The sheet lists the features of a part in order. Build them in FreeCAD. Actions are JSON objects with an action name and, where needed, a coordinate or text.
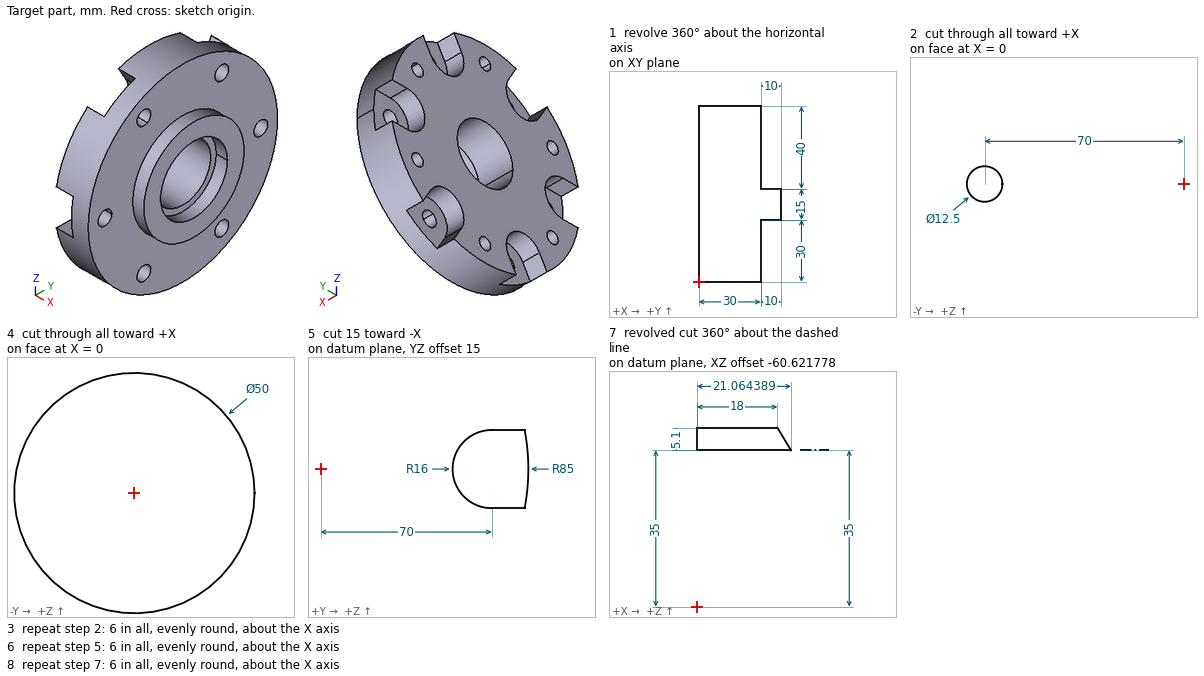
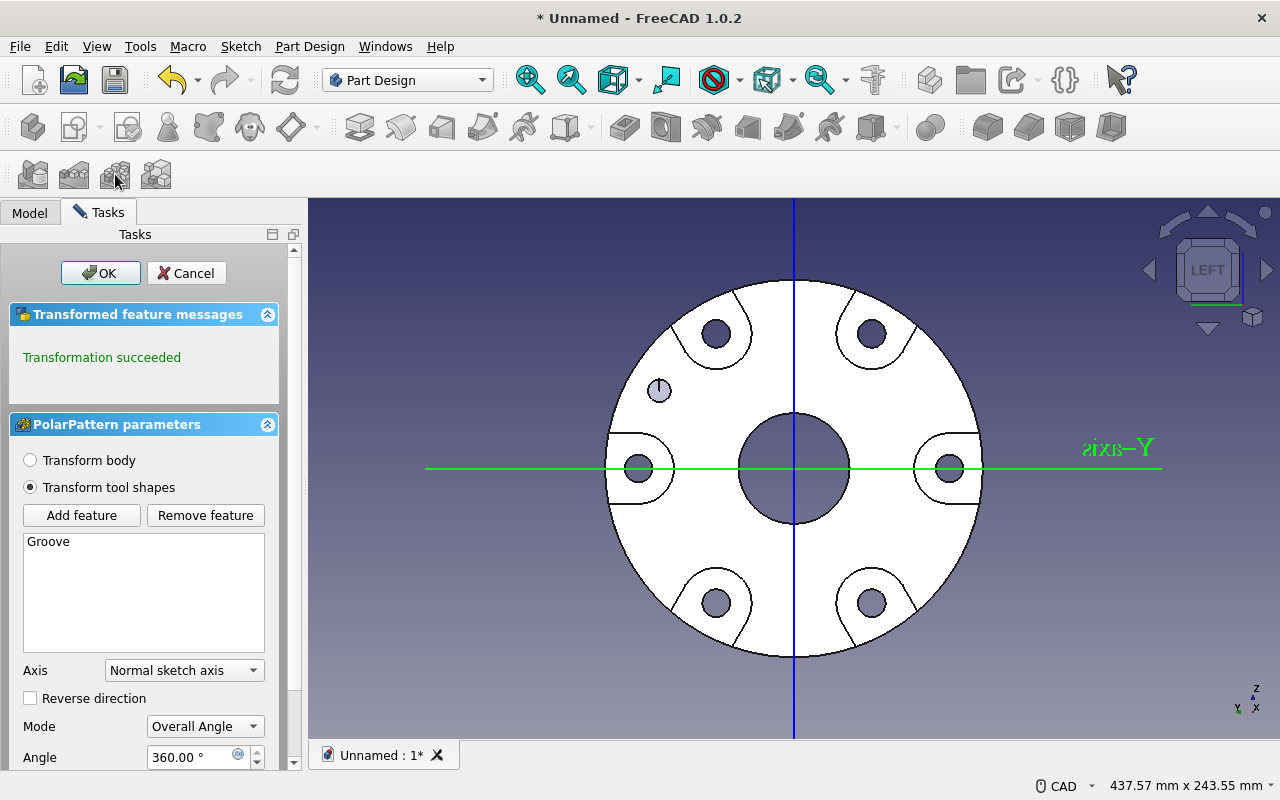
{"action": "left_click", "coordinate": [185, 670]}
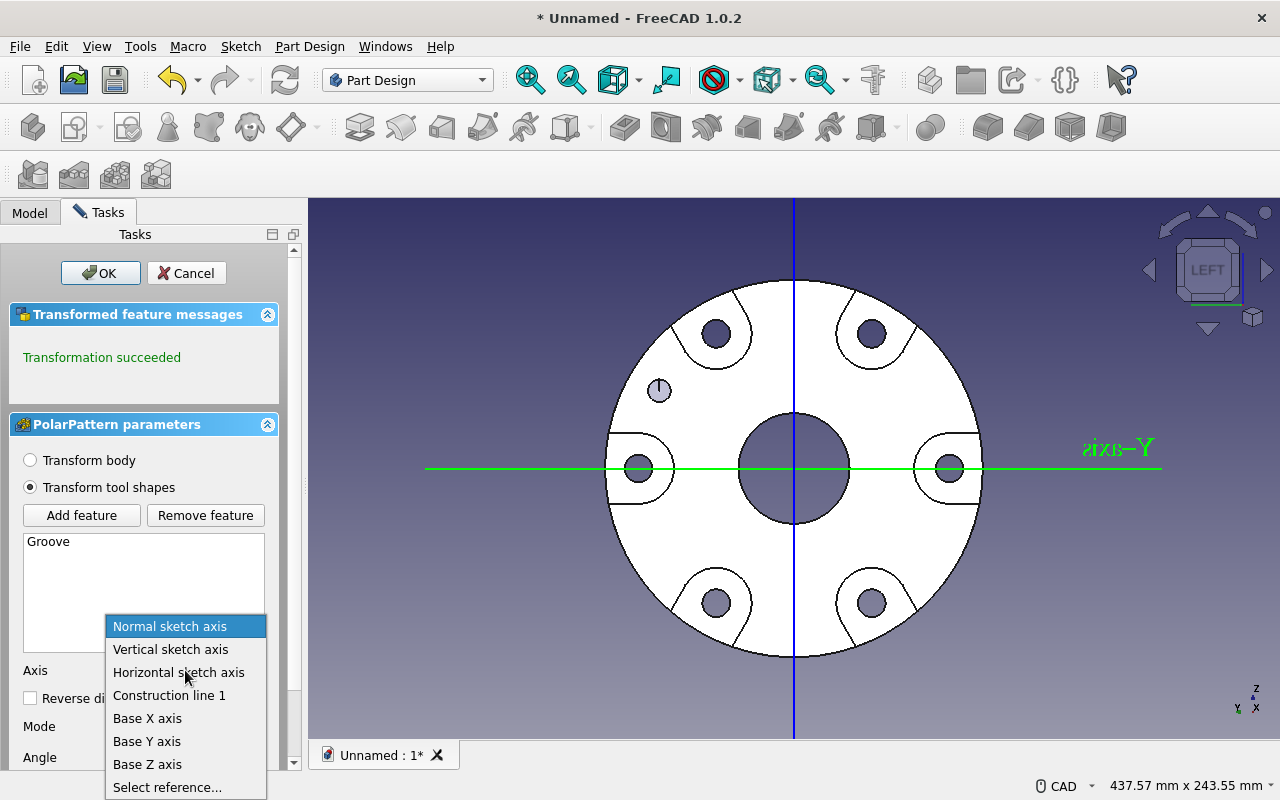
{"action": "left_click", "coordinate": [184, 718]}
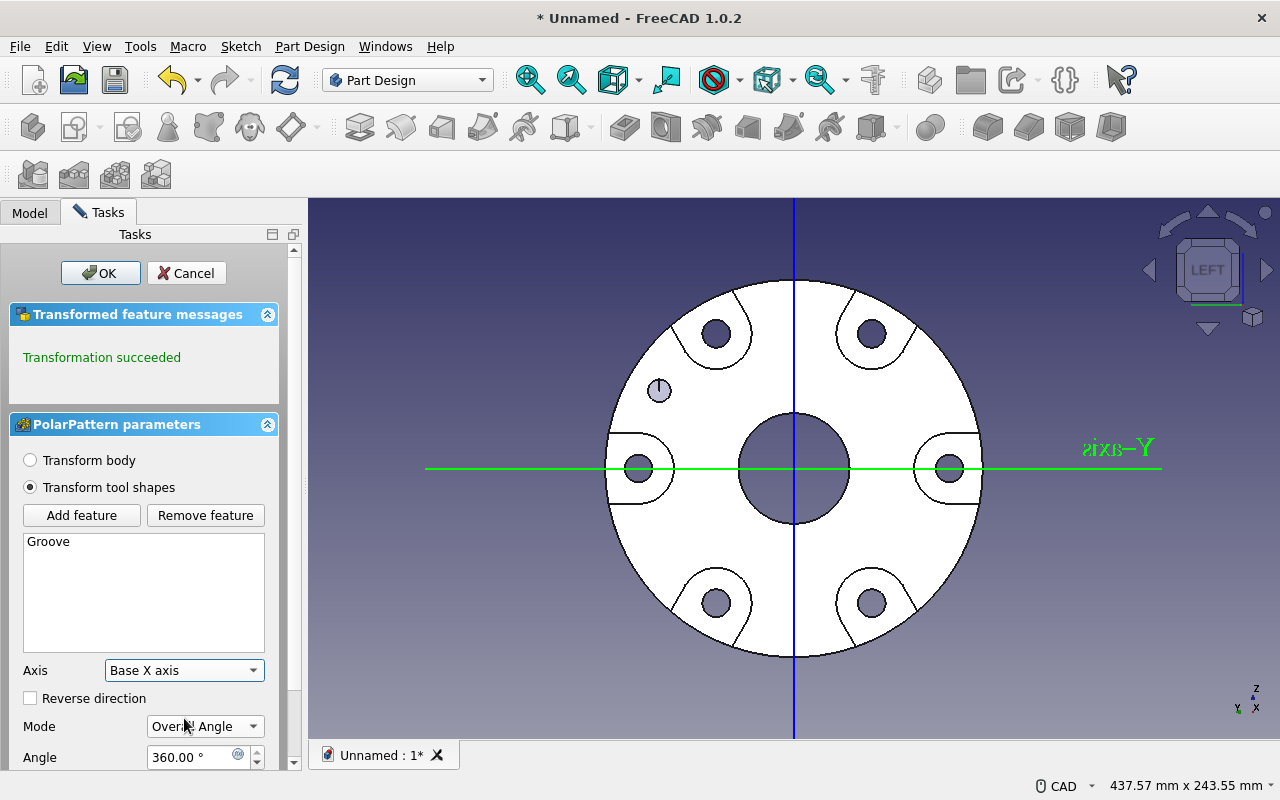
{"action": "scroll", "coordinate": [294, 507], "scroll_direction": "down", "scroll_amount": 2}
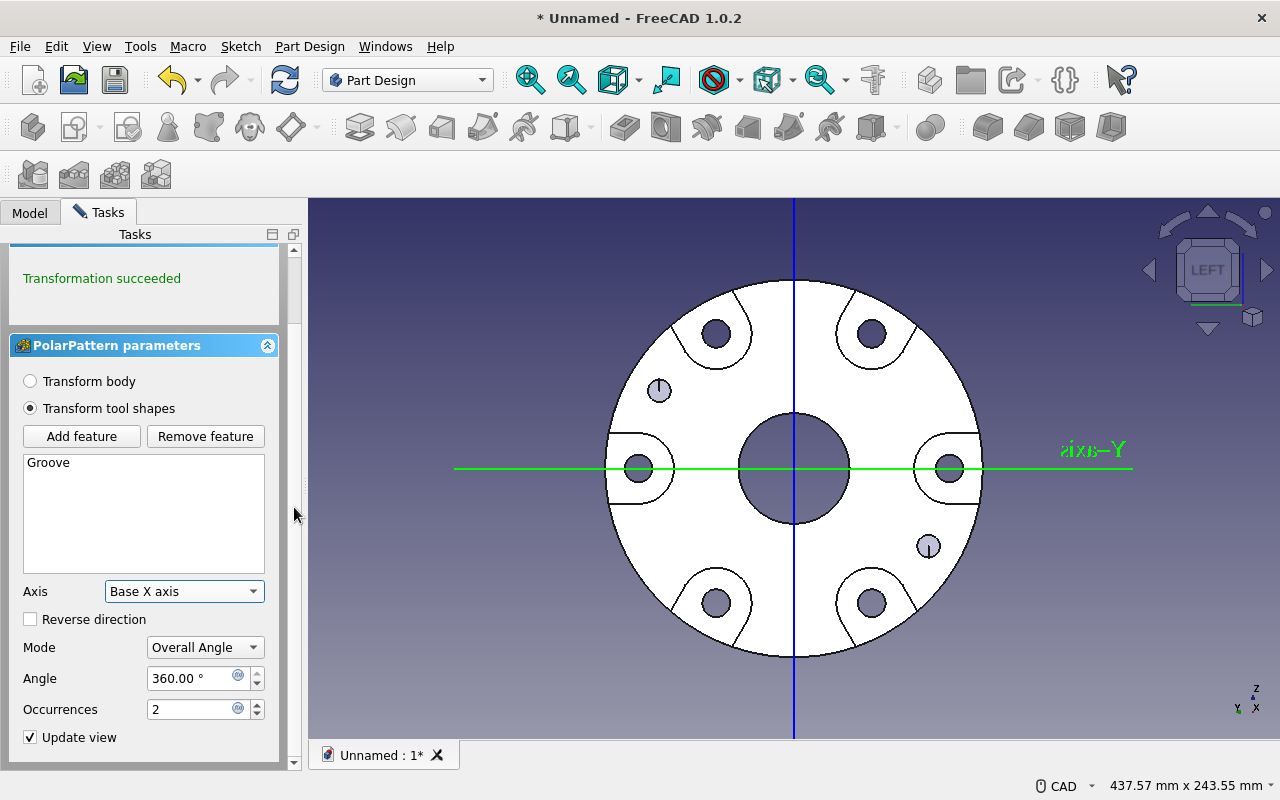
{"action": "triple_click", "coordinate": [199, 710]}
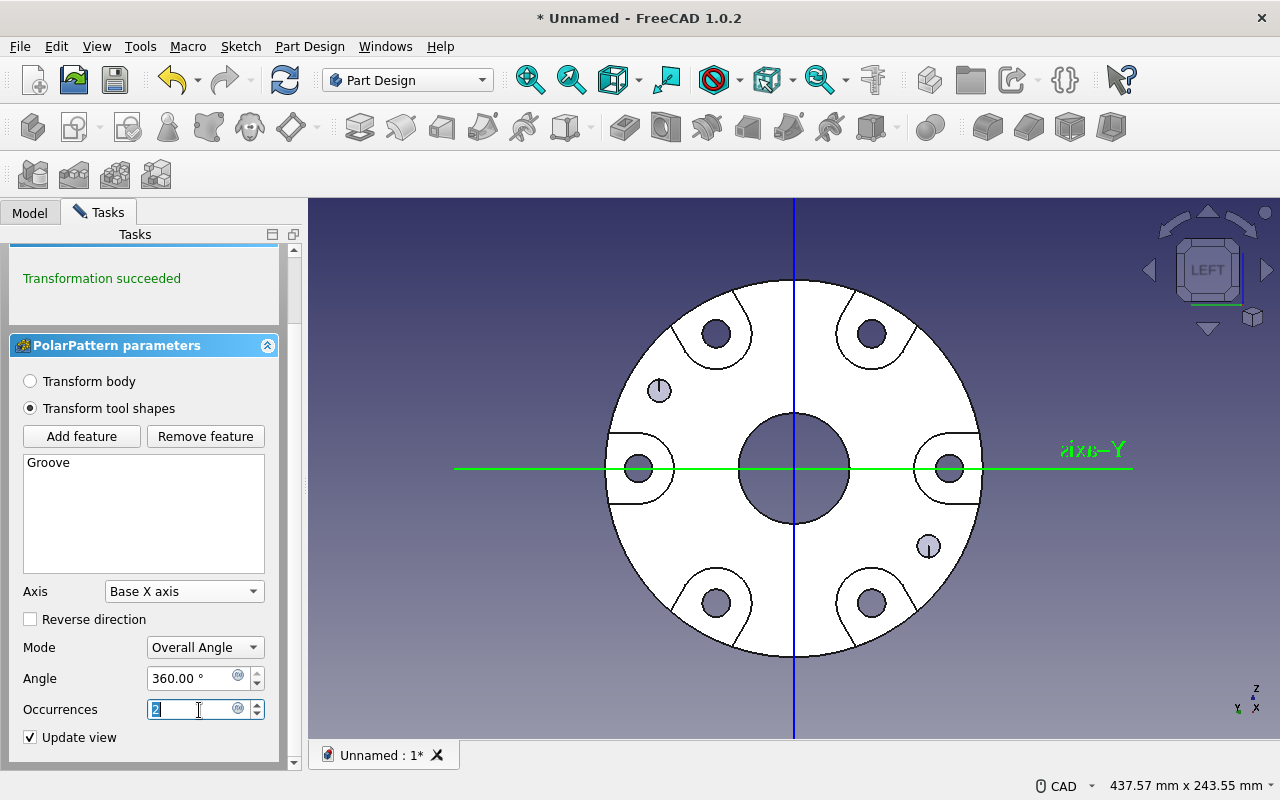
{"action": "type", "text": "6"}
{"action": "key", "text": "Tab"}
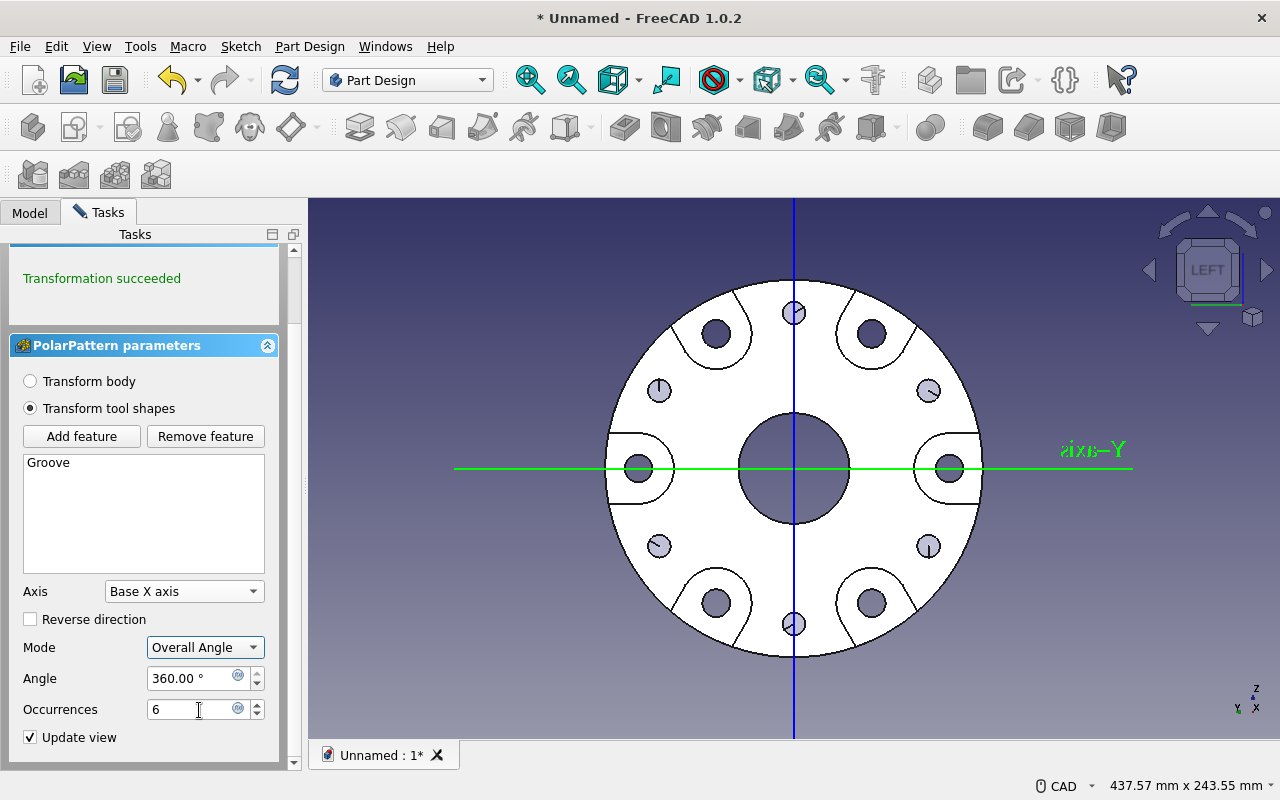
{"action": "scroll", "coordinate": [294, 507], "scroll_direction": "up", "scroll_amount": 3}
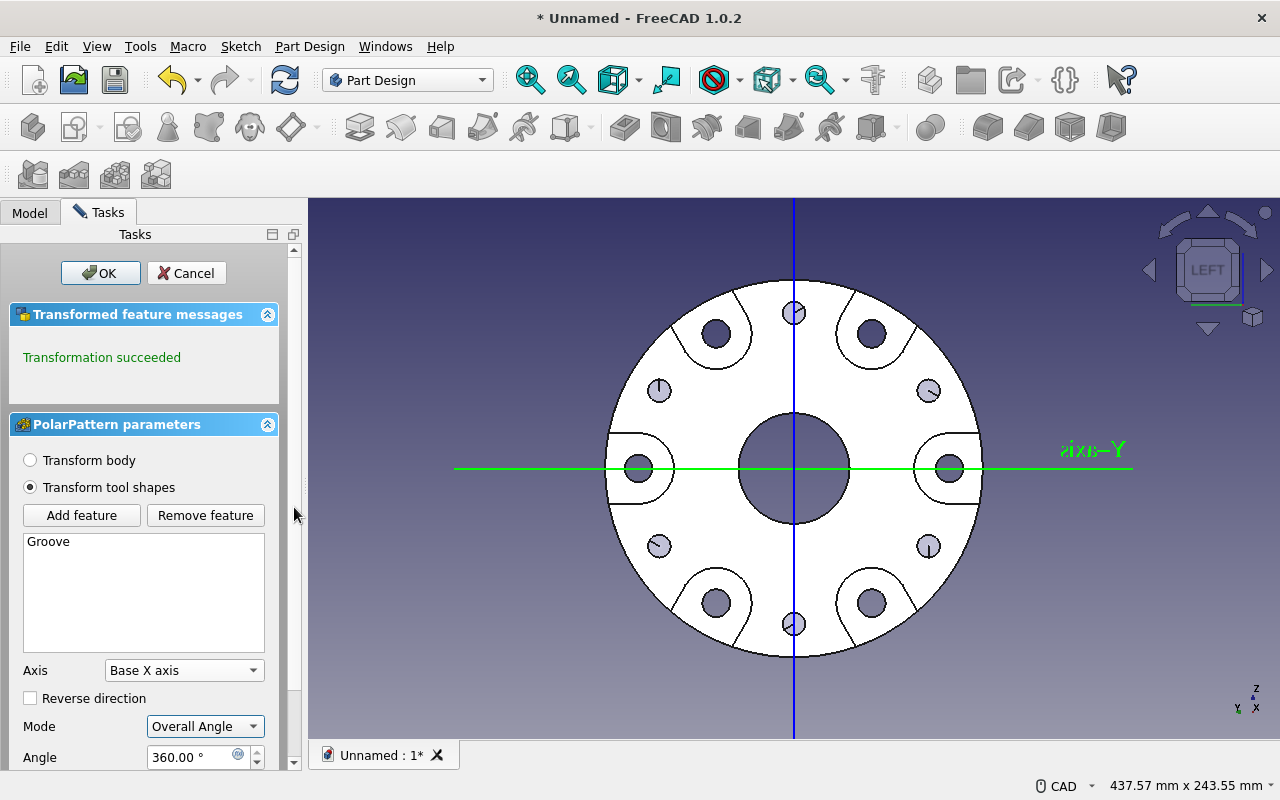
{"action": "left_click", "coordinate": [101, 273]}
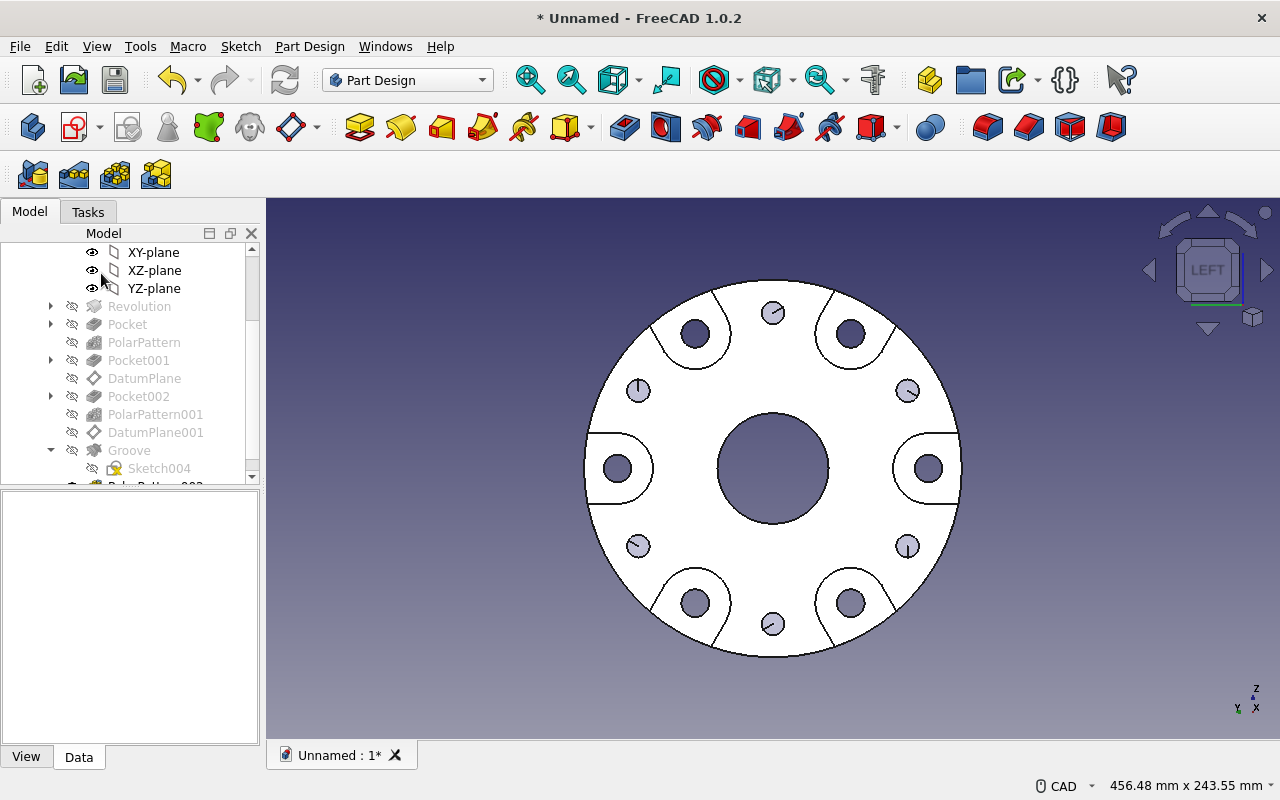
{"action": "key", "text": "0"}